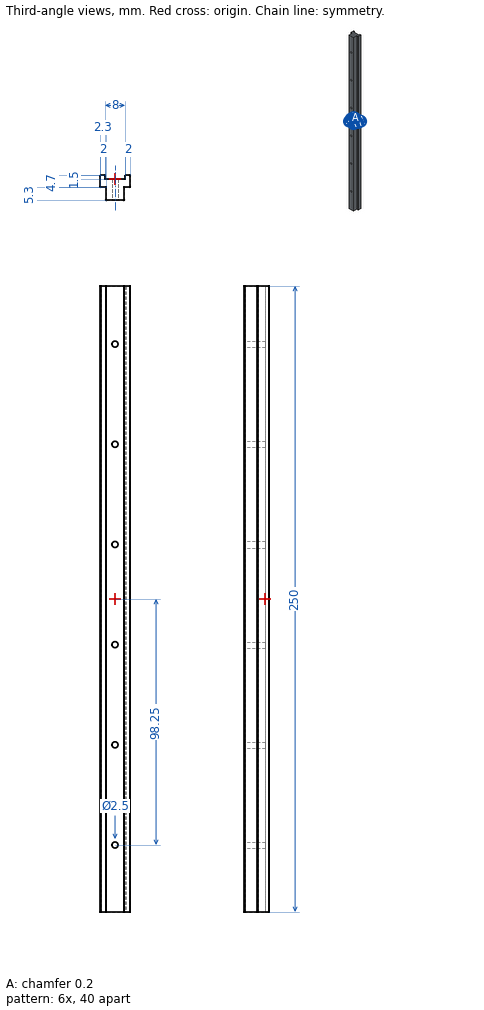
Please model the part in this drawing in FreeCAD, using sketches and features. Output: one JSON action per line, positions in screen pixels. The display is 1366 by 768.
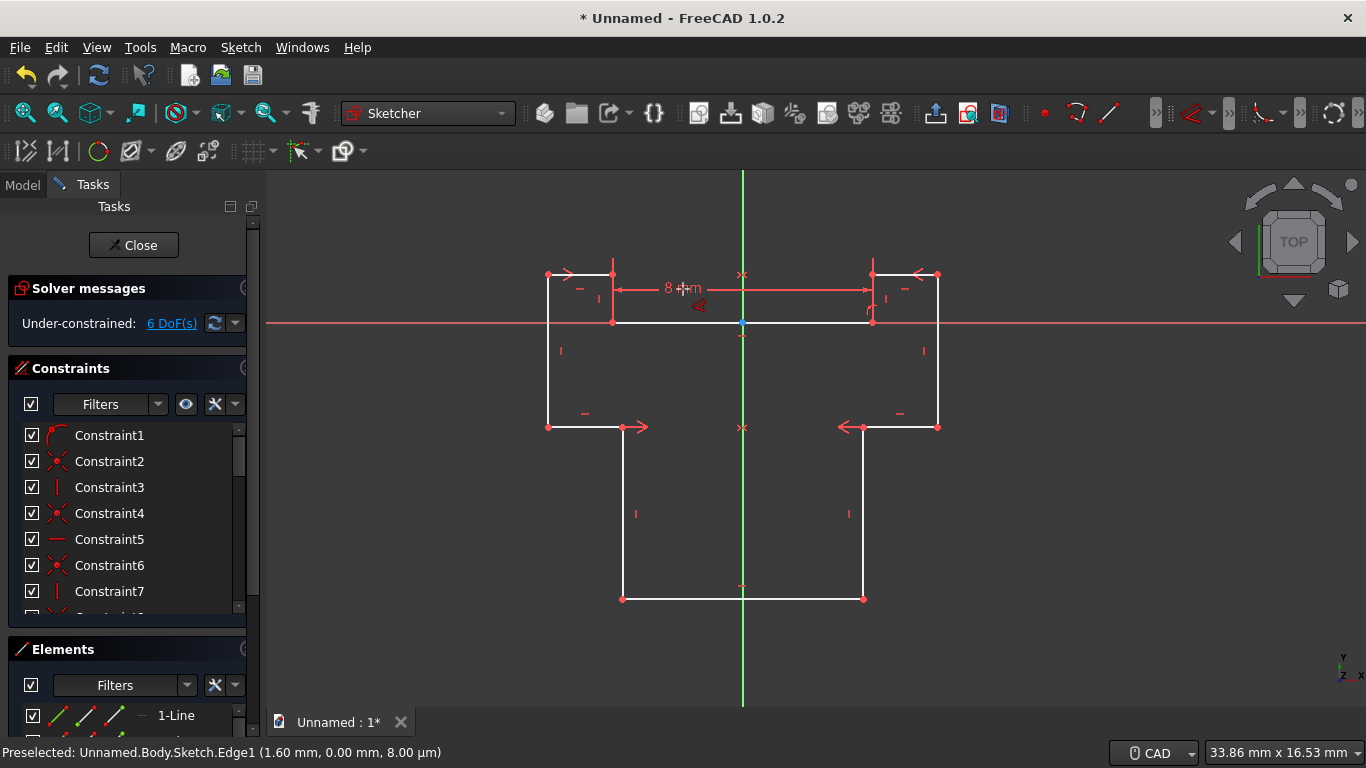
{"action": "left_click", "coordinate": [593, 275]}
{"action": "left_click", "coordinate": [581, 241]}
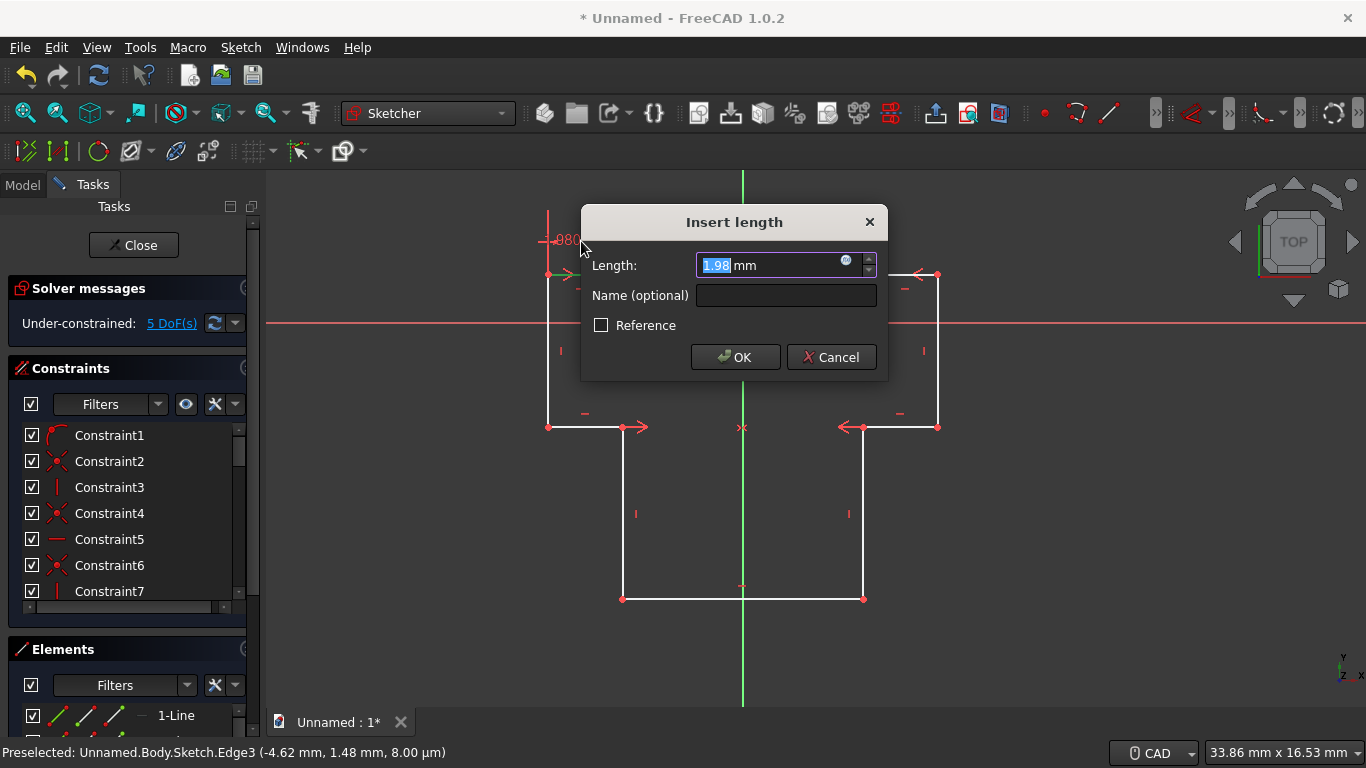
{"action": "type", "text": "2"}
{"action": "key", "text": "Return"}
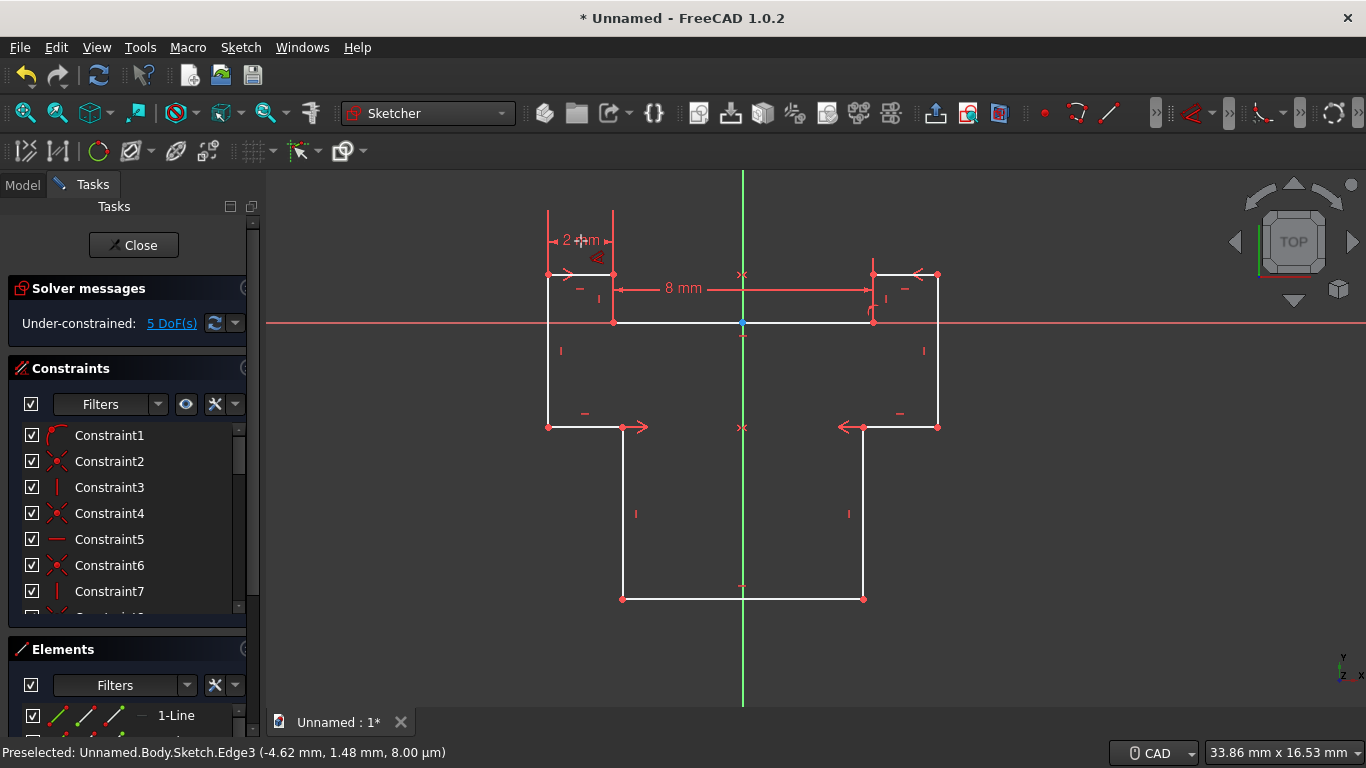
{"action": "left_click", "coordinate": [918, 275]}
{"action": "left_click", "coordinate": [905, 241]}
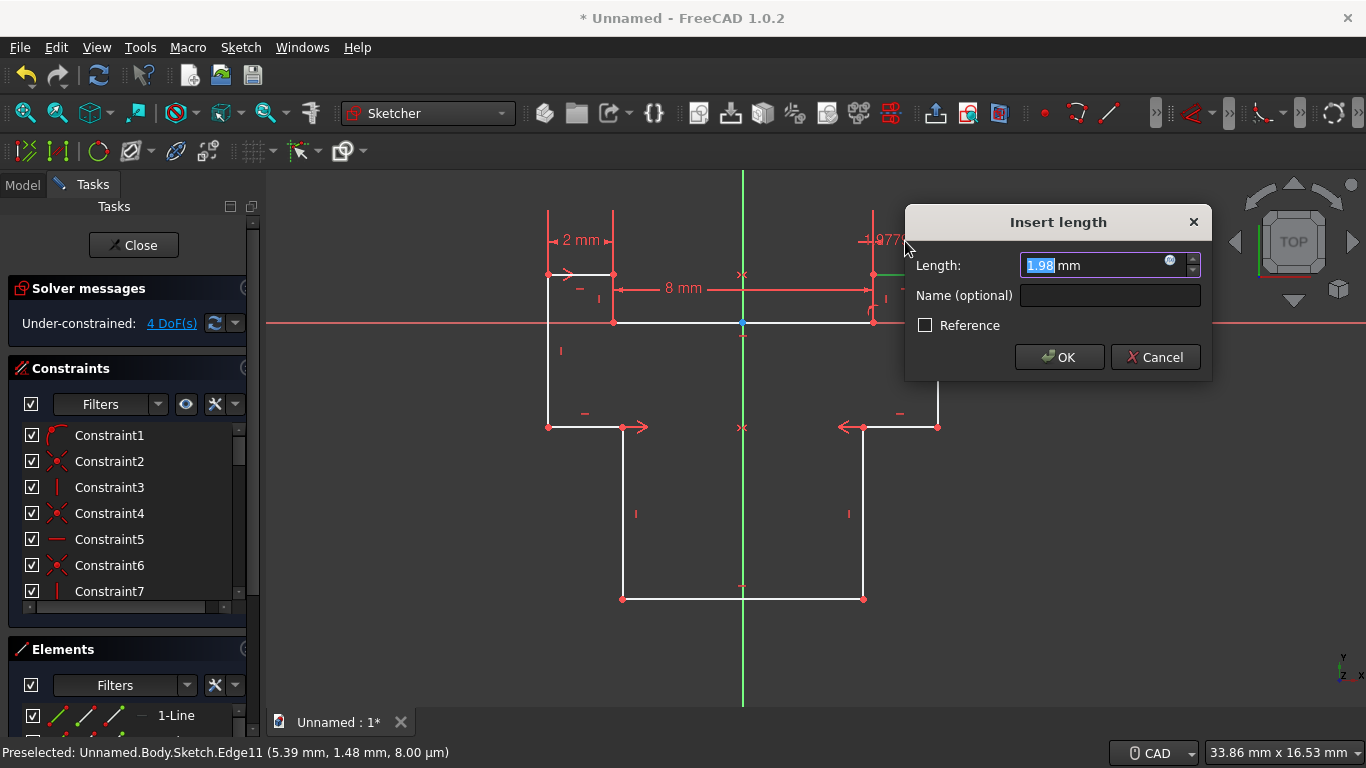
{"action": "type", "text": "2"}
{"action": "key", "text": "Return"}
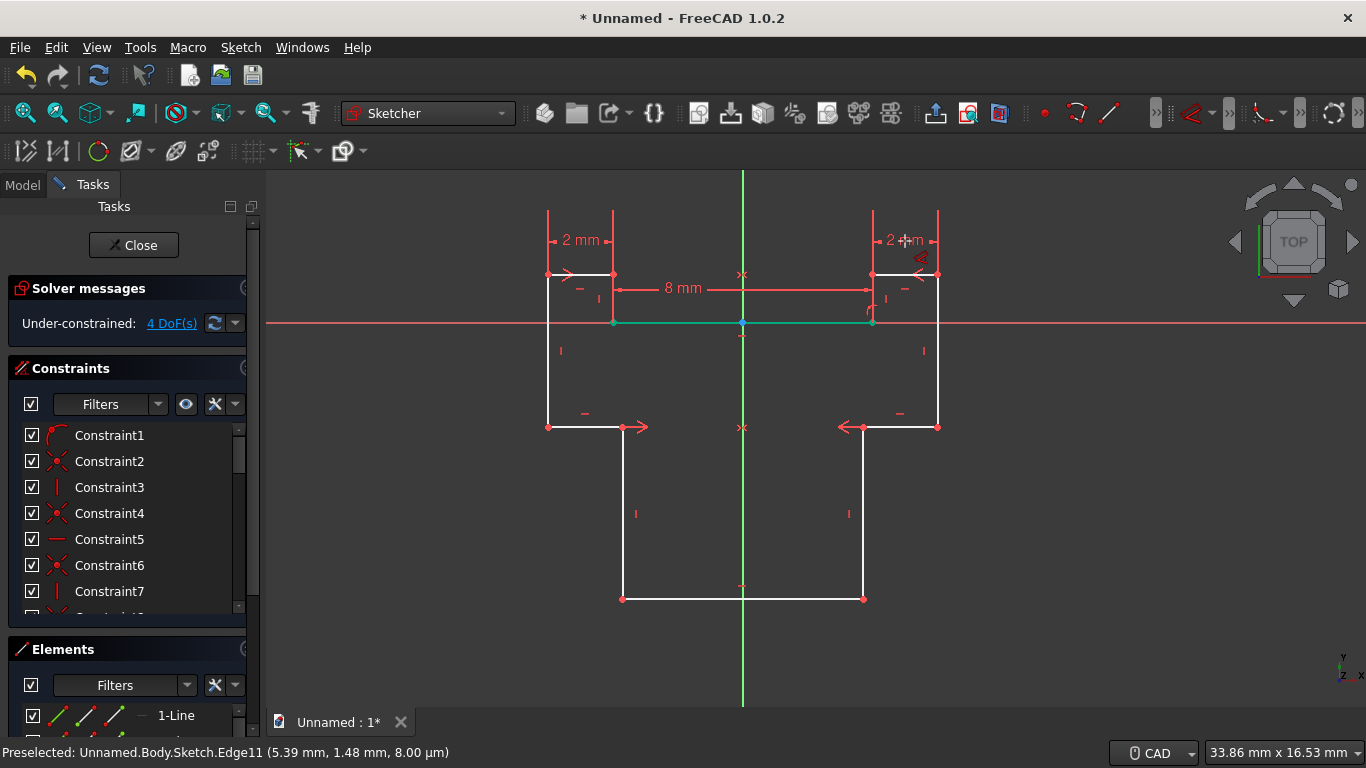
{"action": "left_click", "coordinate": [613, 308]}
{"action": "left_click", "coordinate": [579, 299]}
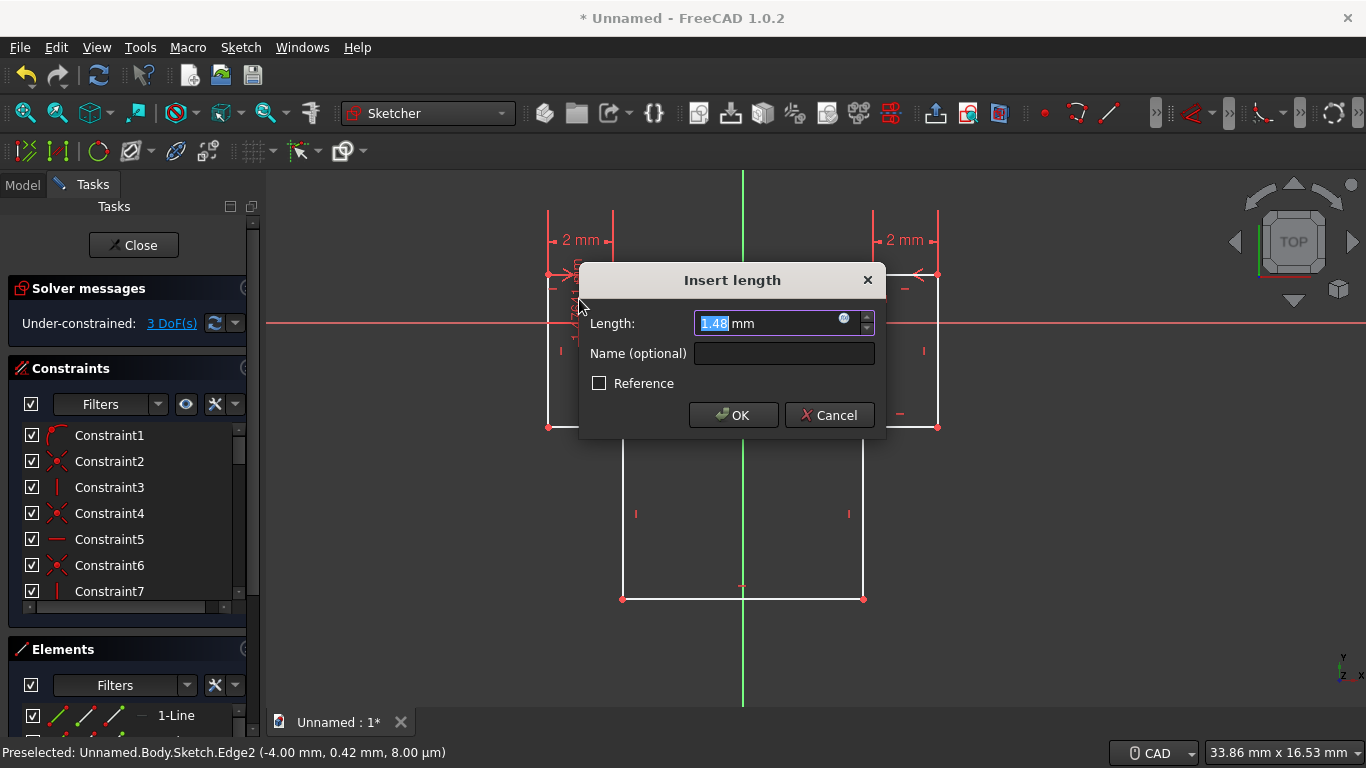
{"action": "type", "text": "1.5"}
{"action": "key", "text": "Return"}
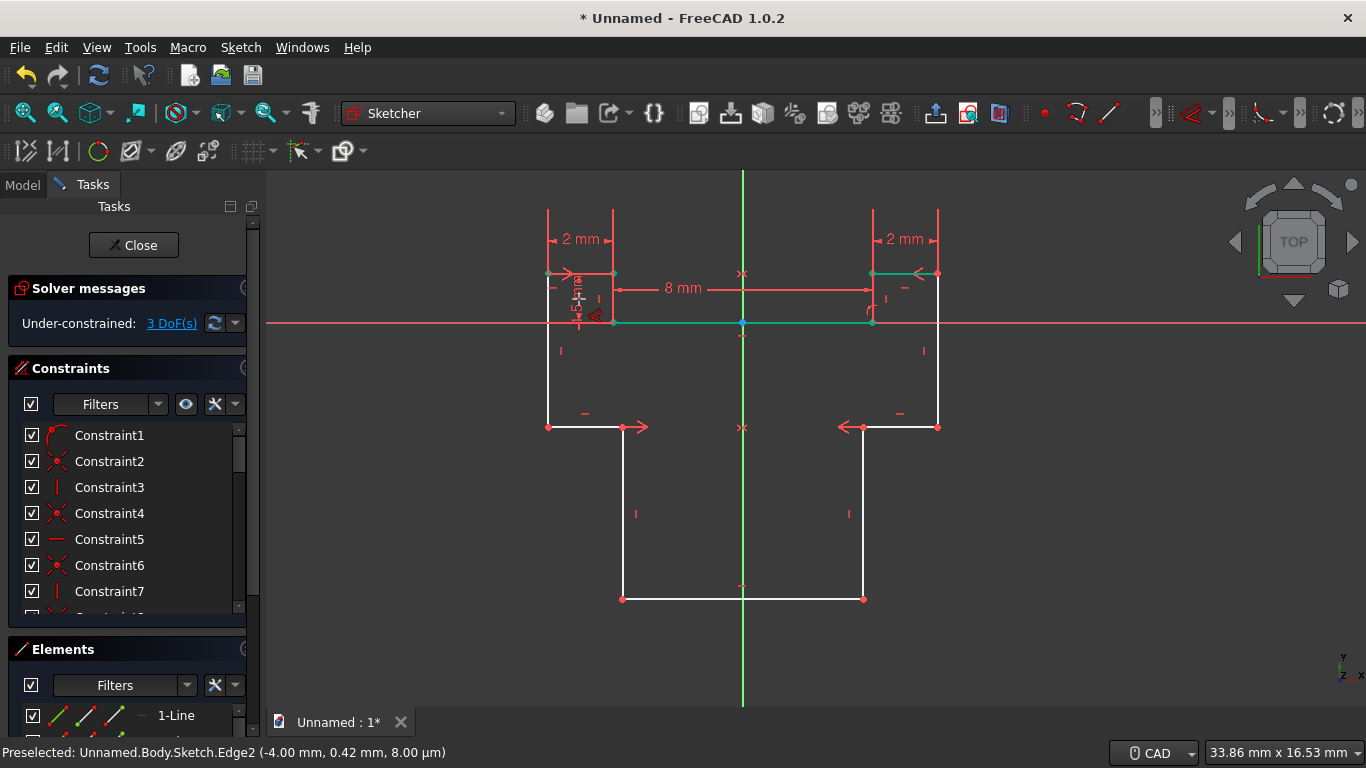
{"action": "left_click", "coordinate": [548, 320]}
{"action": "left_click", "coordinate": [514, 350]}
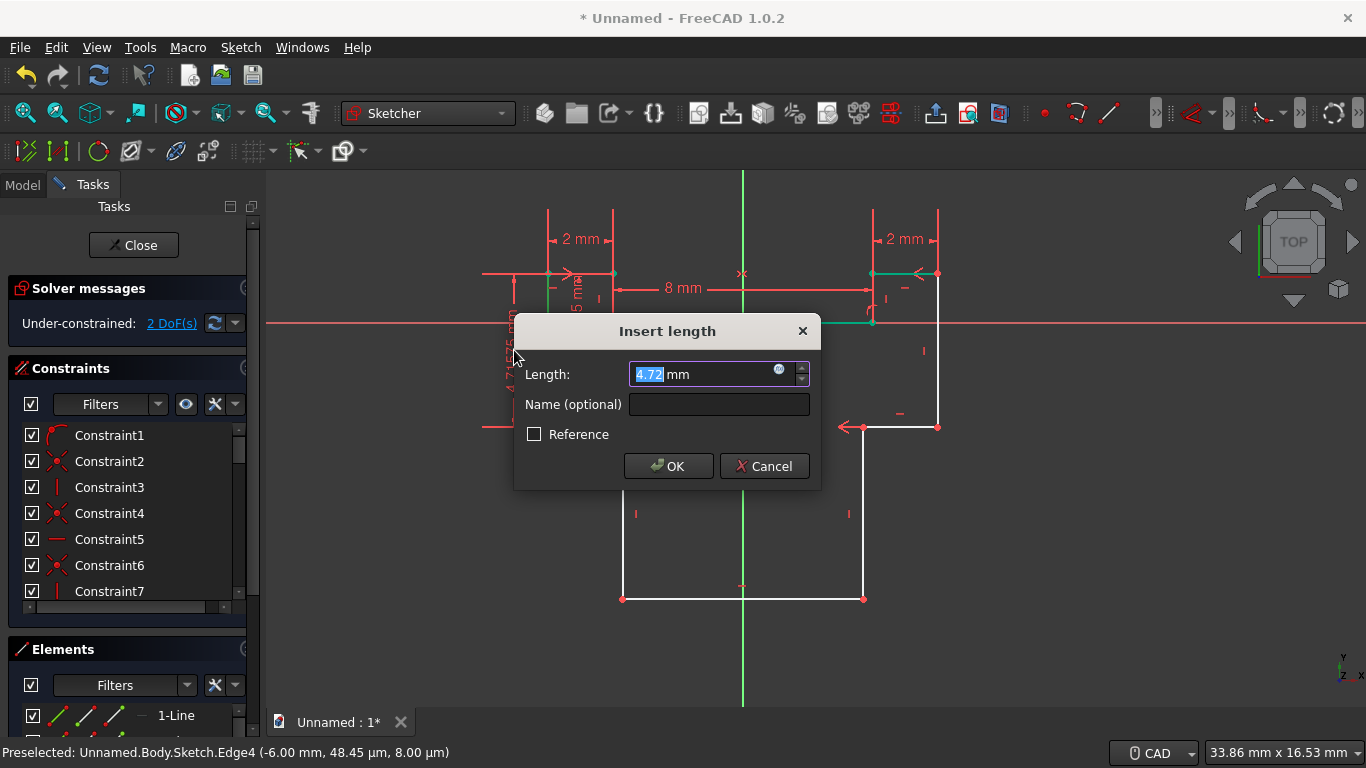
{"action": "type", "text": "4.7"}
{"action": "key", "text": "Return"}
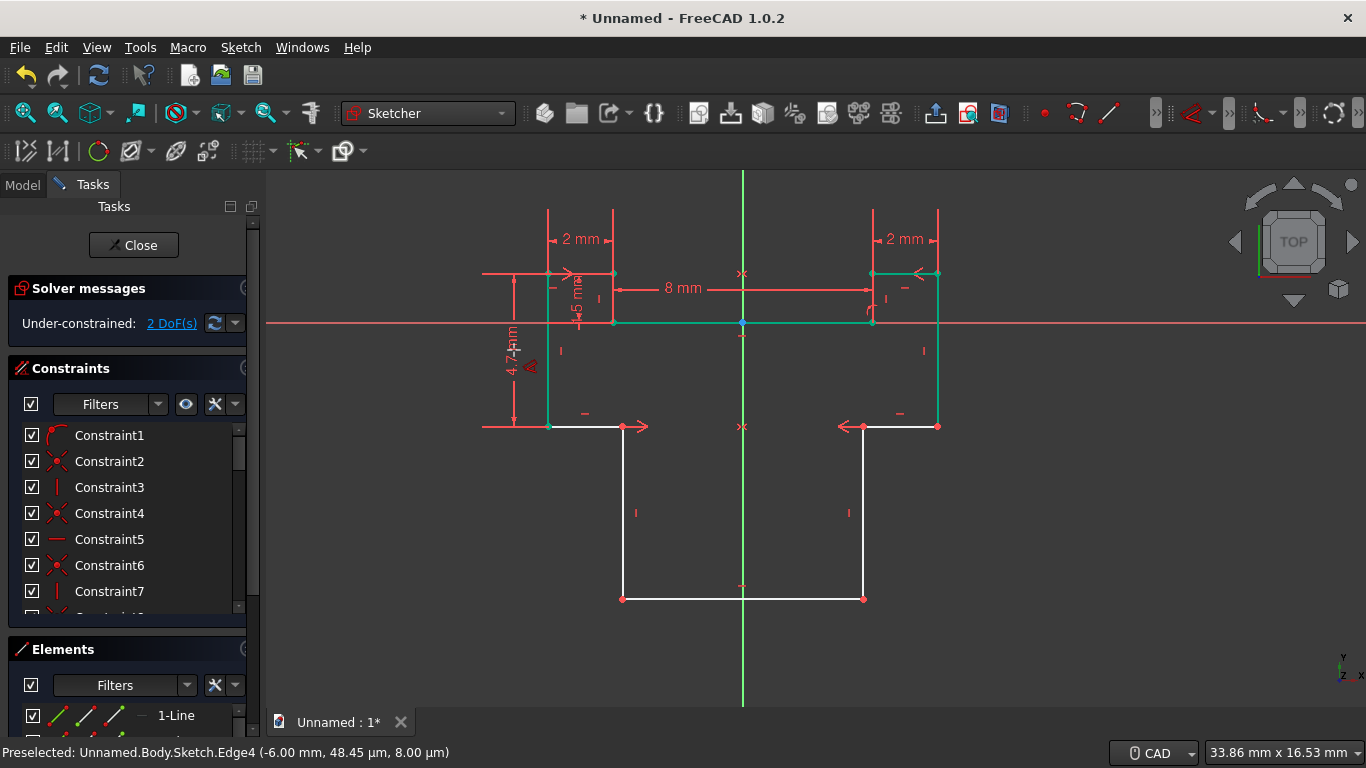
{"action": "left_click", "coordinate": [570, 427]}
{"action": "left_click", "coordinate": [585, 393]}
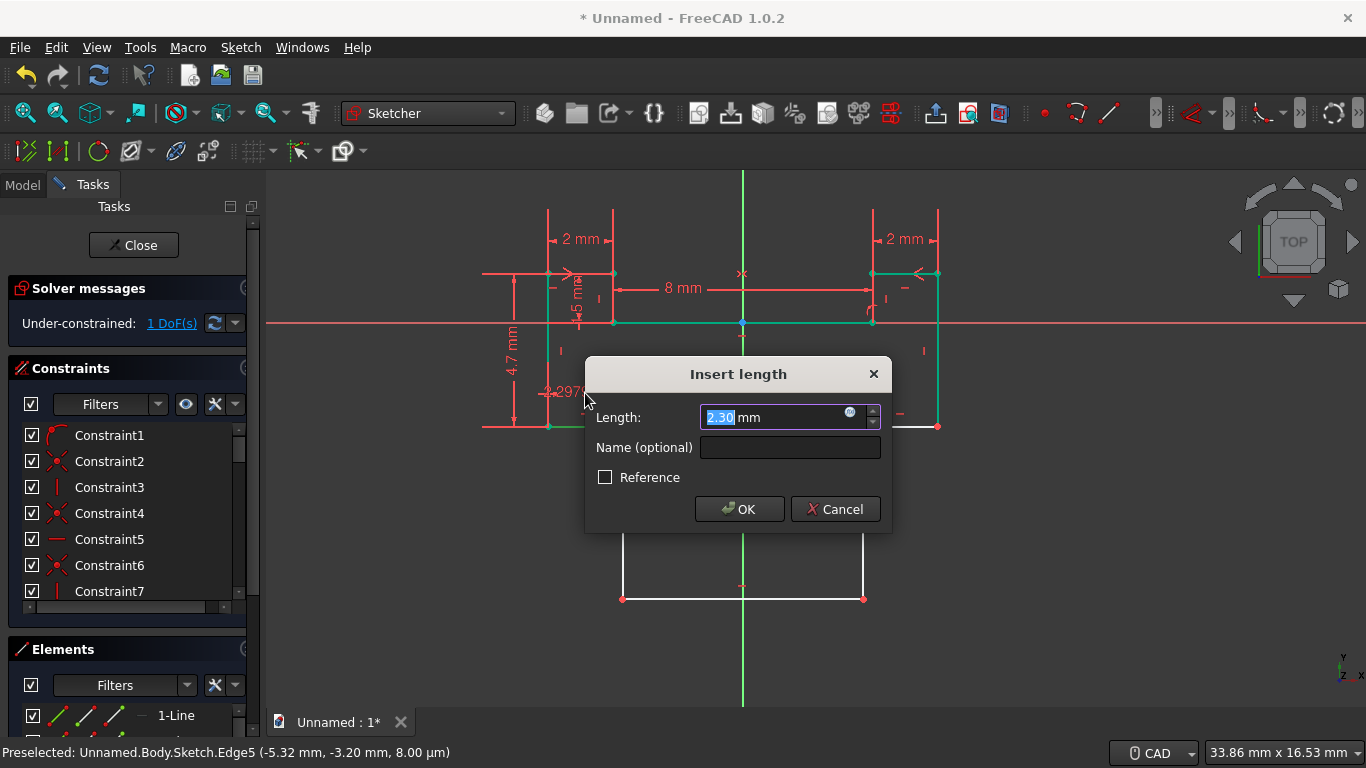
{"action": "type", "text": "2.3"}
{"action": "key", "text": "Return"}